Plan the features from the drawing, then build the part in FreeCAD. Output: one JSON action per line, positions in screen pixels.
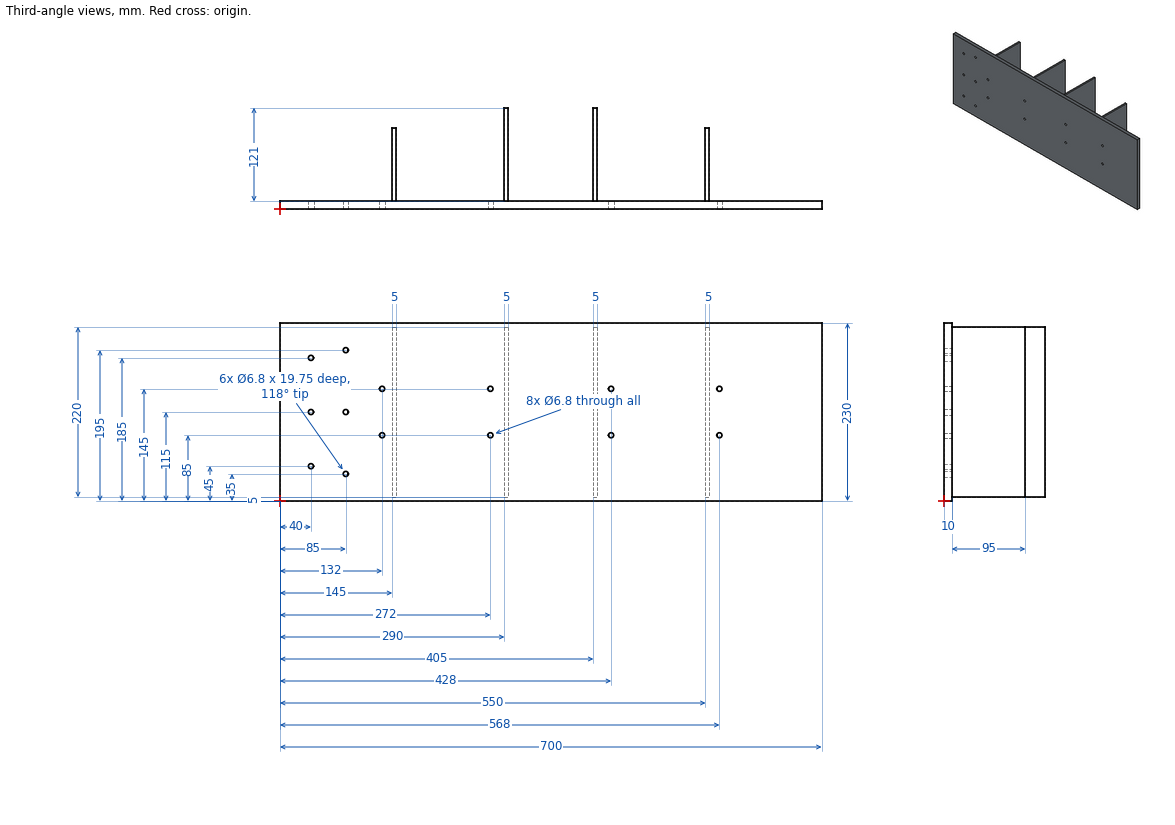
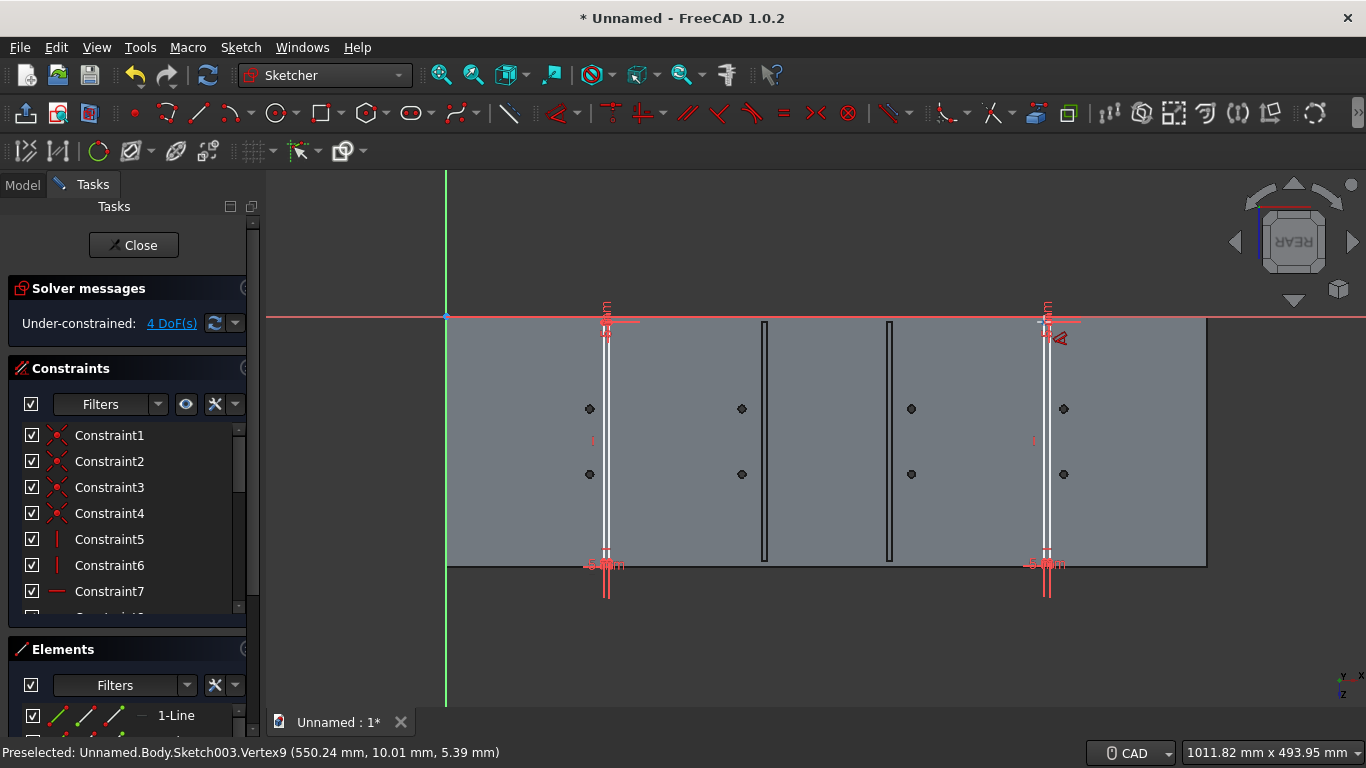
{"action": "scroll", "coordinate": [604, 394], "scroll_direction": "up", "scroll_amount": 5}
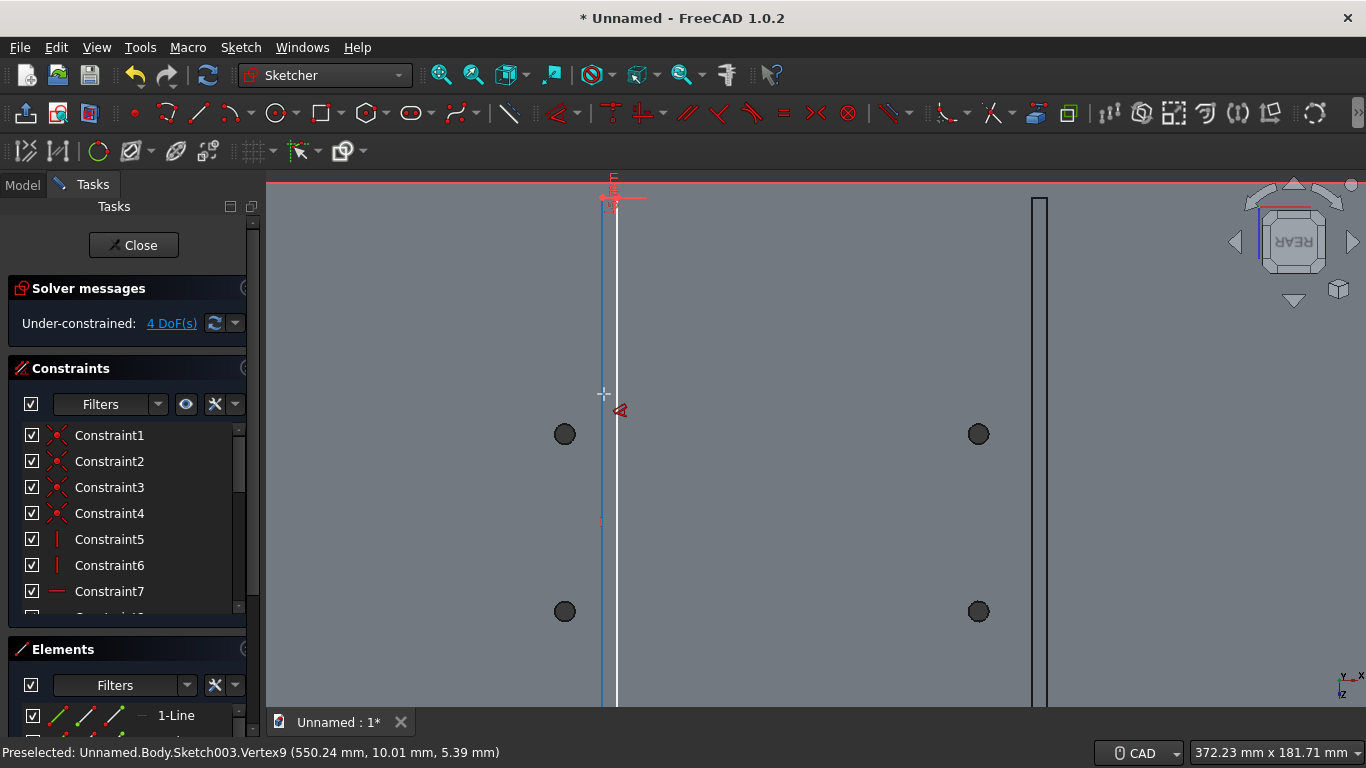
{"action": "left_click", "coordinate": [602, 393]}
{"action": "left_click", "coordinate": [568, 438]}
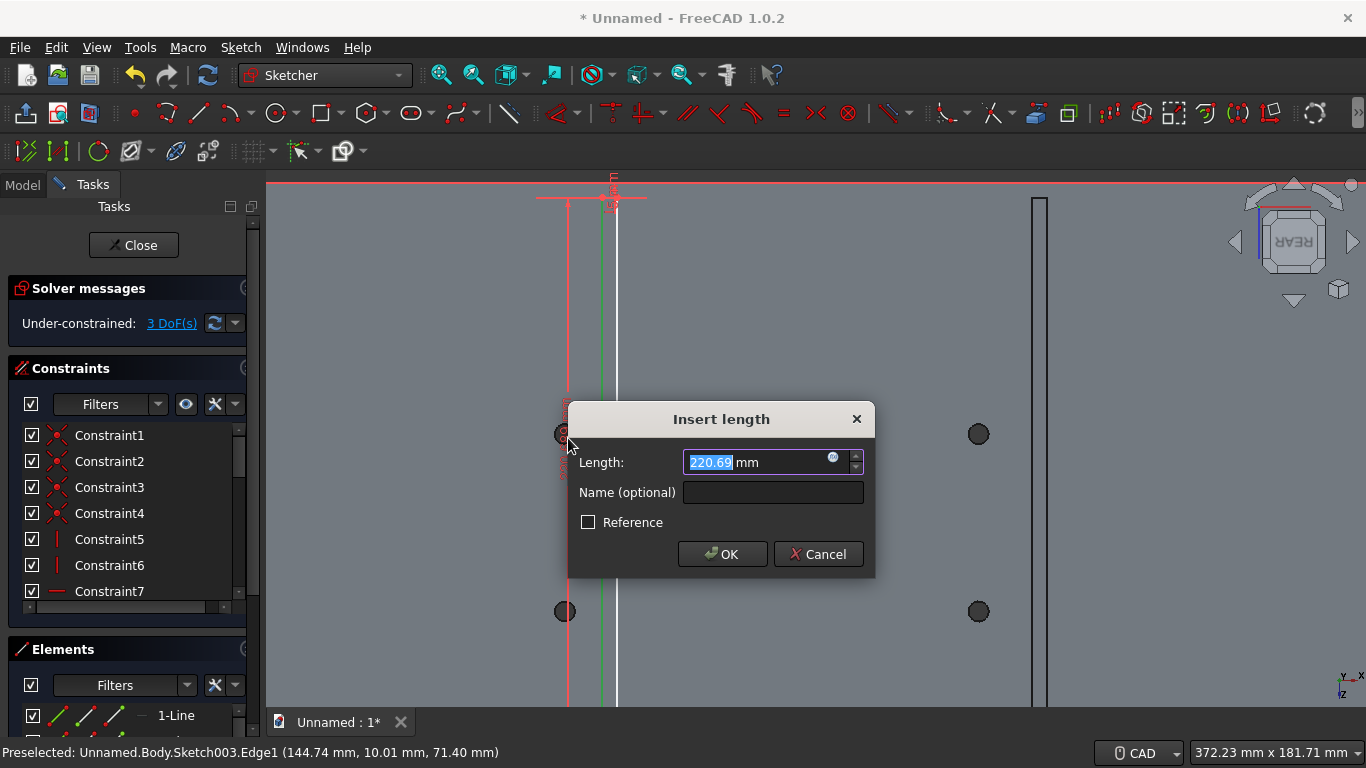
{"action": "type", "text": "220"}
{"action": "key", "text": "Return"}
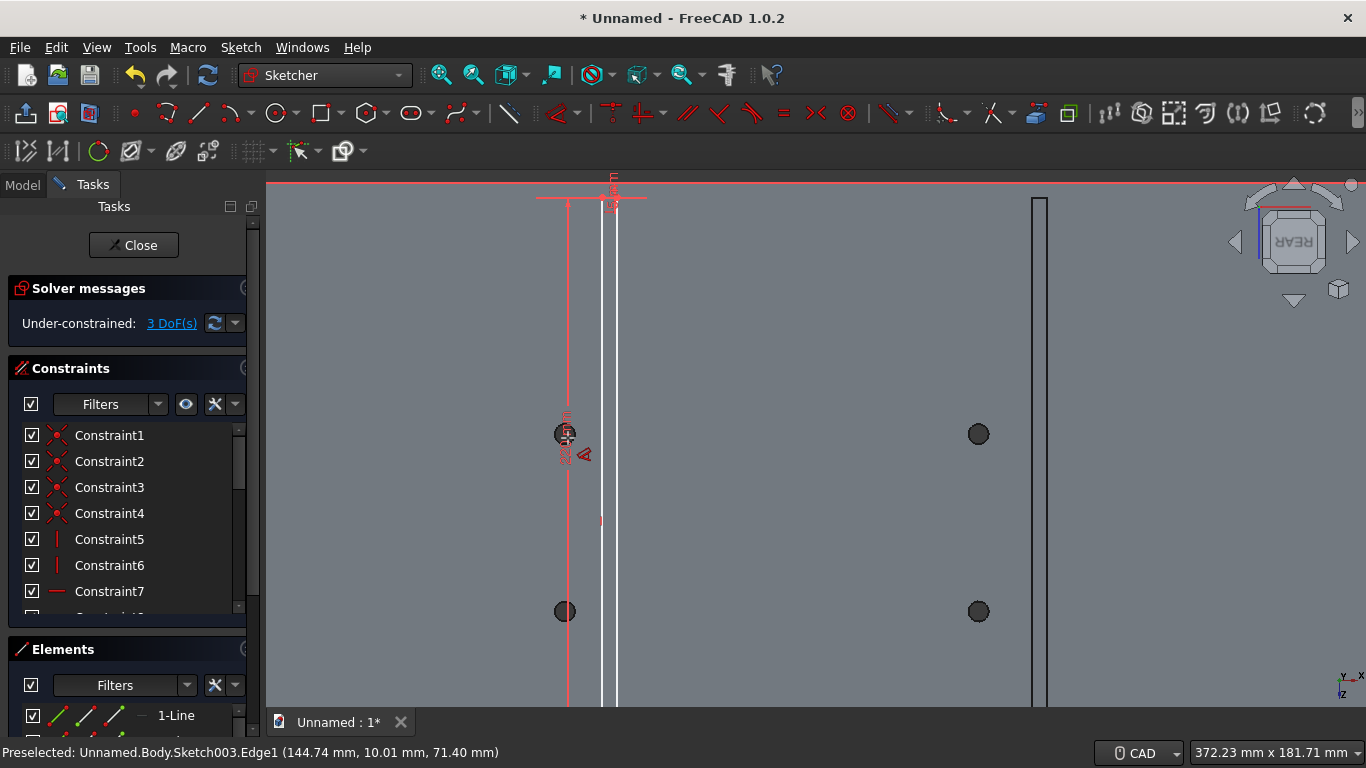
{"action": "scroll", "coordinate": [604, 394], "scroll_direction": "down", "scroll_amount": 5}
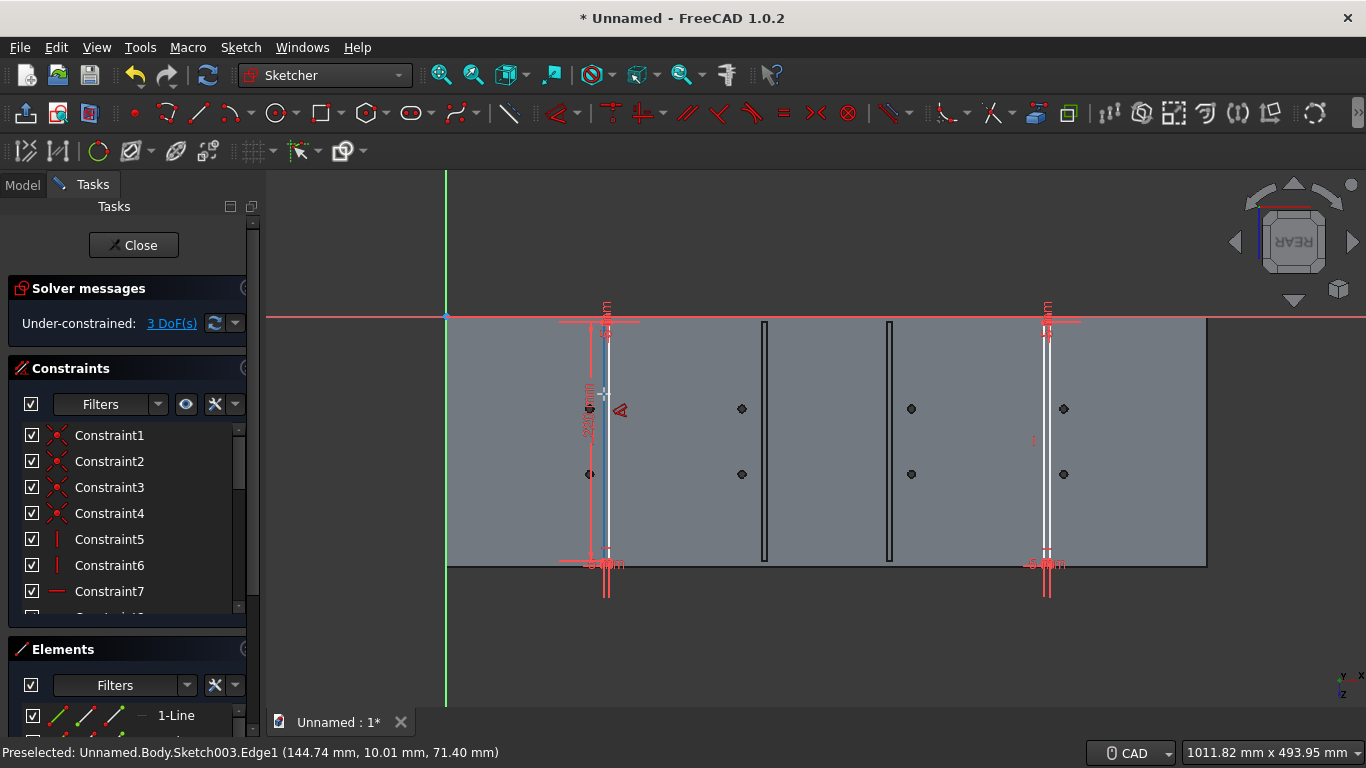
{"action": "scroll", "coordinate": [1044, 394], "scroll_direction": "up", "scroll_amount": 5}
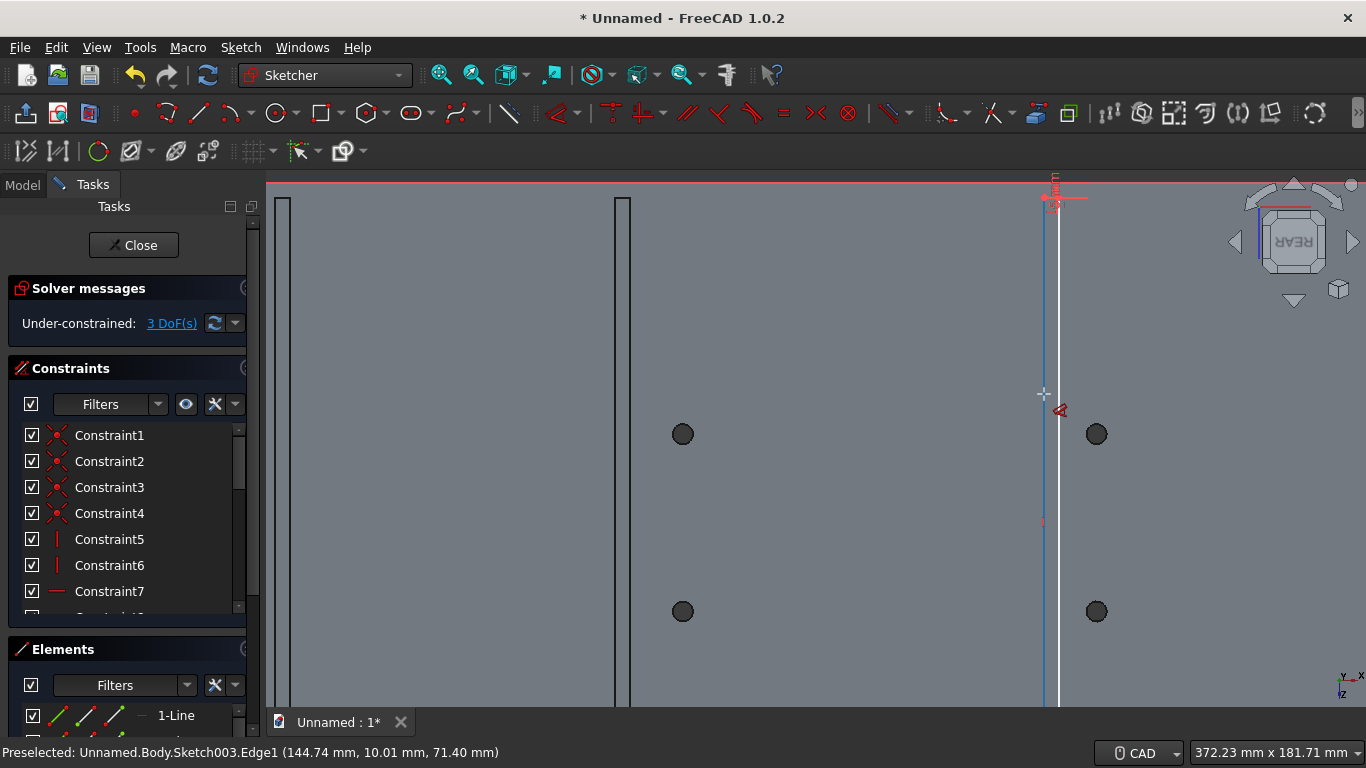
{"action": "left_click", "coordinate": [1044, 393]}
{"action": "left_click", "coordinate": [1078, 438]}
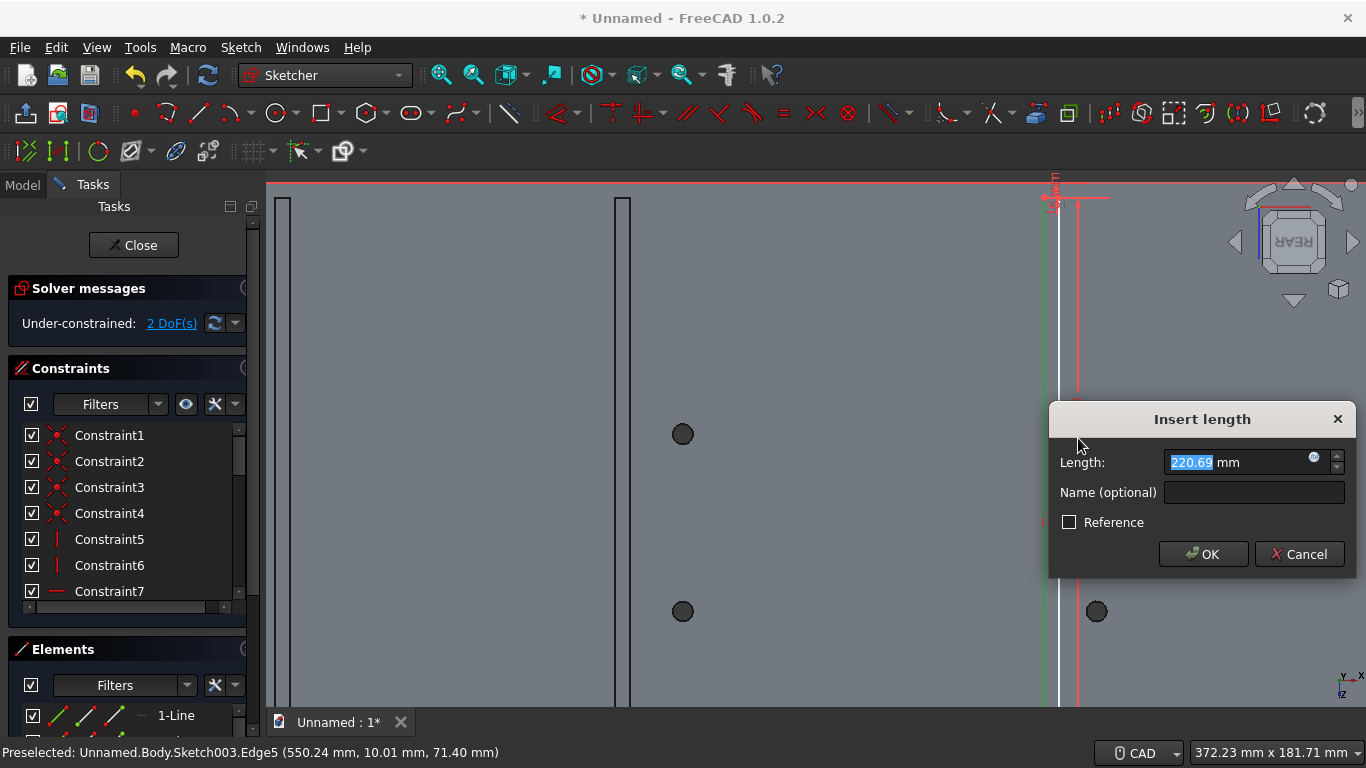
{"action": "type", "text": "220"}
{"action": "key", "text": "Return"}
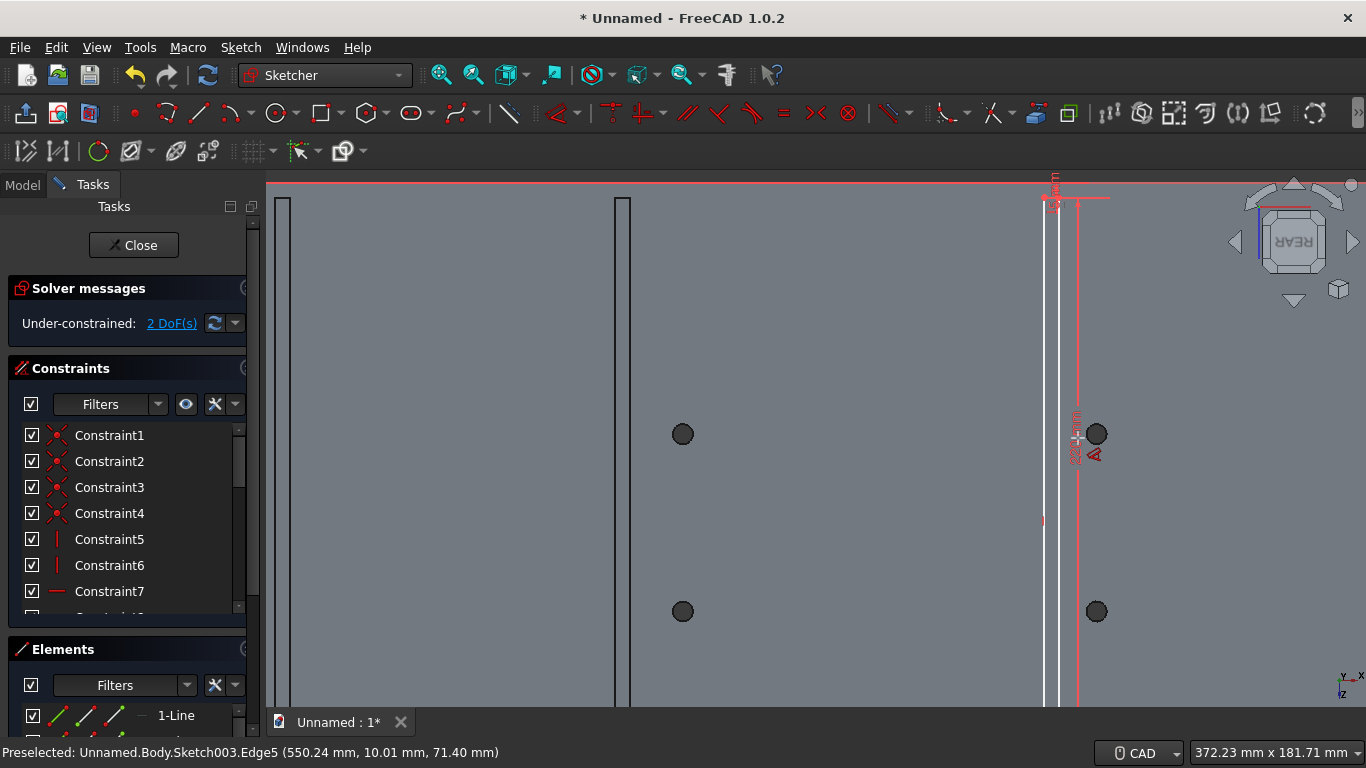
{"action": "scroll", "coordinate": [1044, 394], "scroll_direction": "down", "scroll_amount": 5}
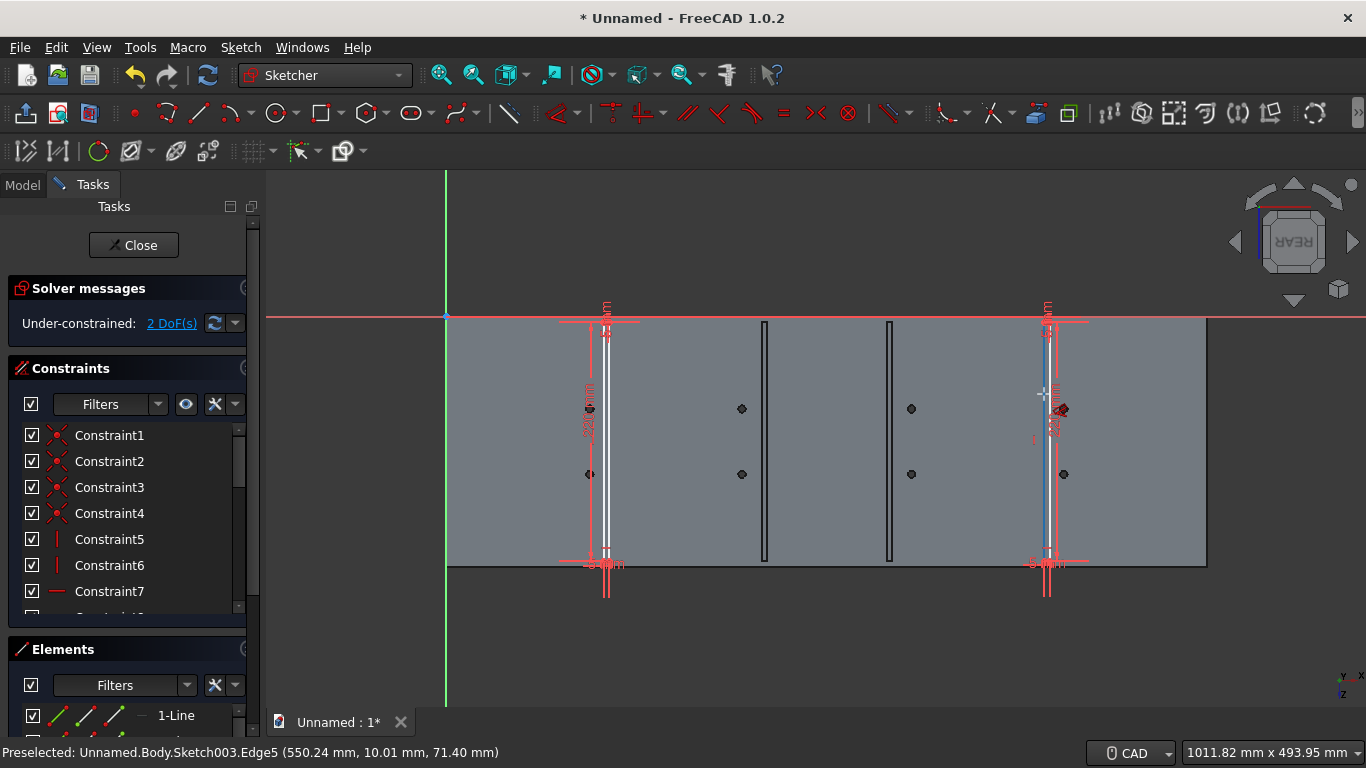
{"action": "scroll", "coordinate": [604, 322], "scroll_direction": "up", "scroll_amount": 5}